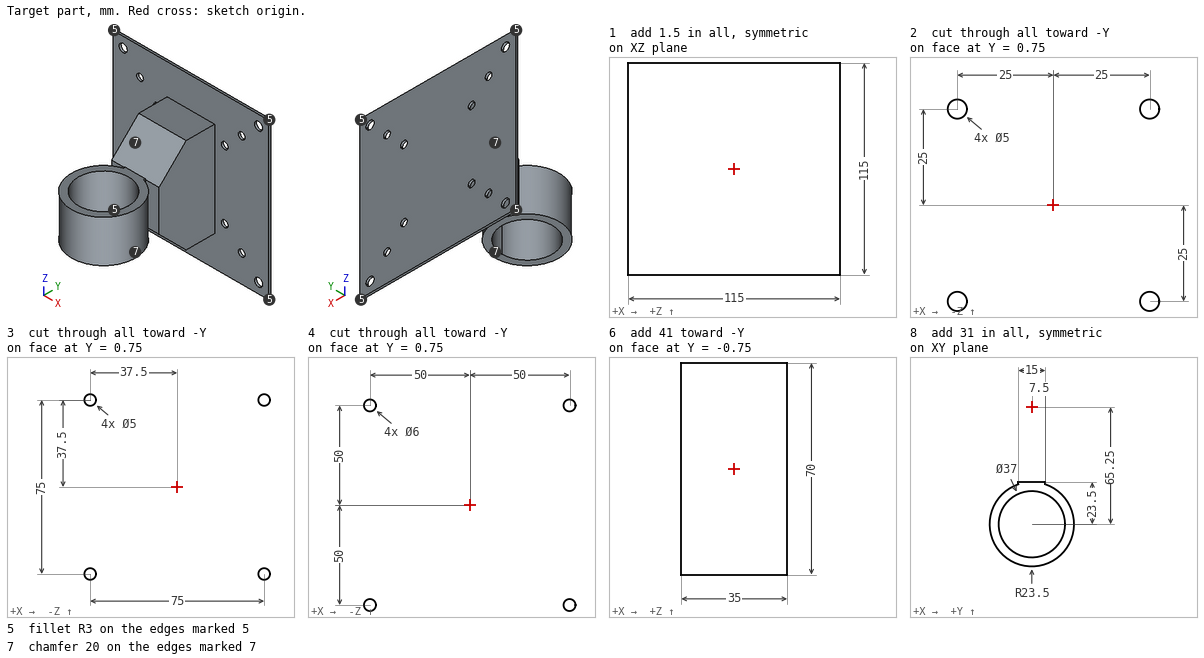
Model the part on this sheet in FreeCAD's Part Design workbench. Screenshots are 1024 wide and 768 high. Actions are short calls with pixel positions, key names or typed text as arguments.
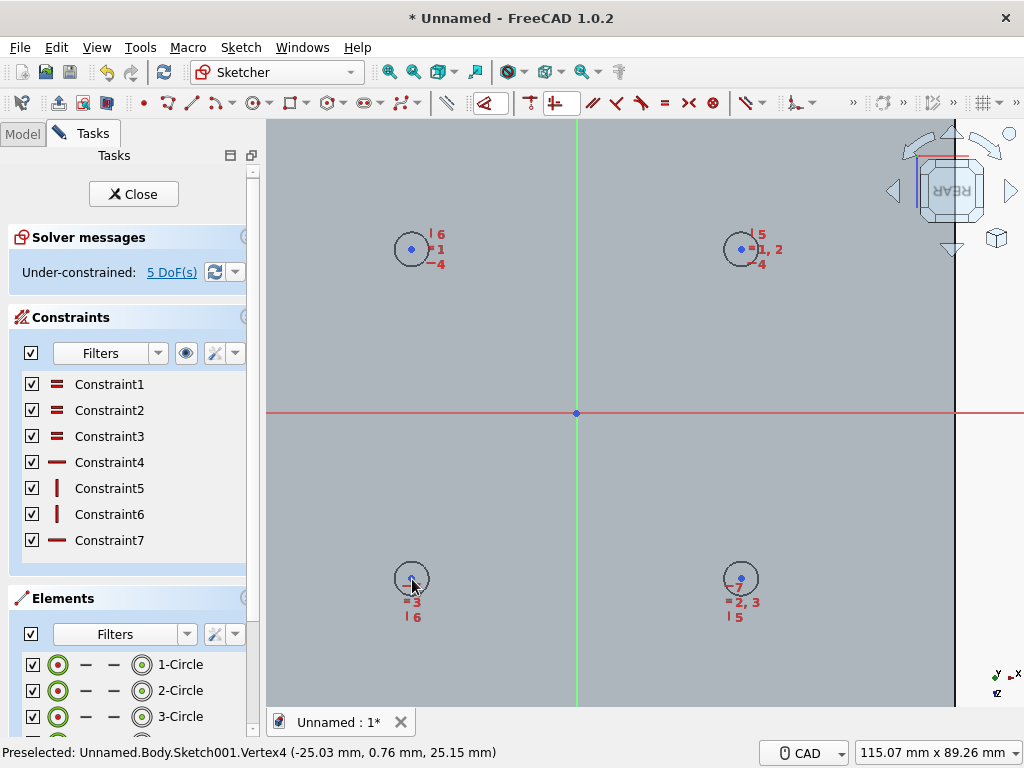
key(d)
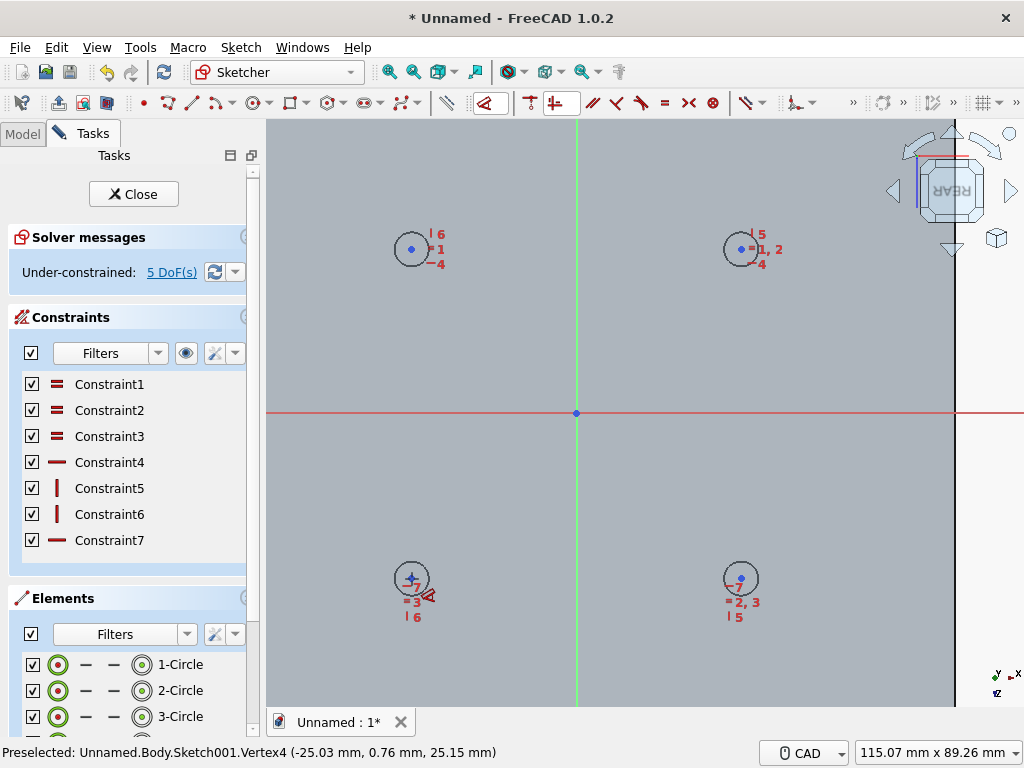
click(424, 237)
click(447, 214)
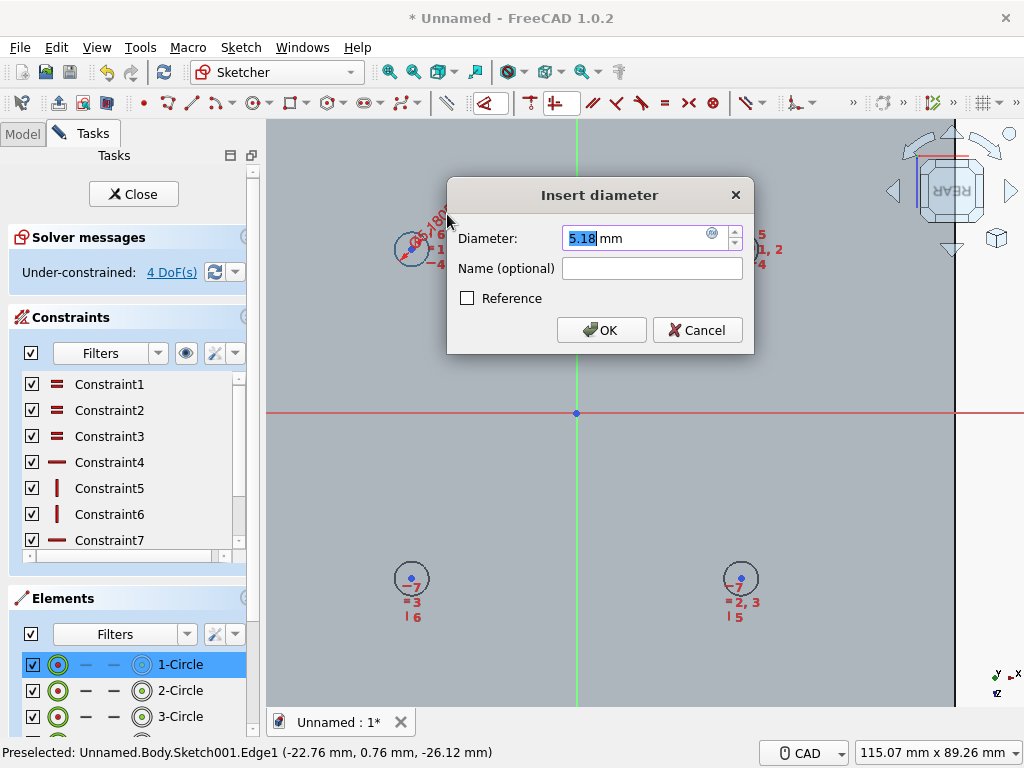
text(5)
key(Return)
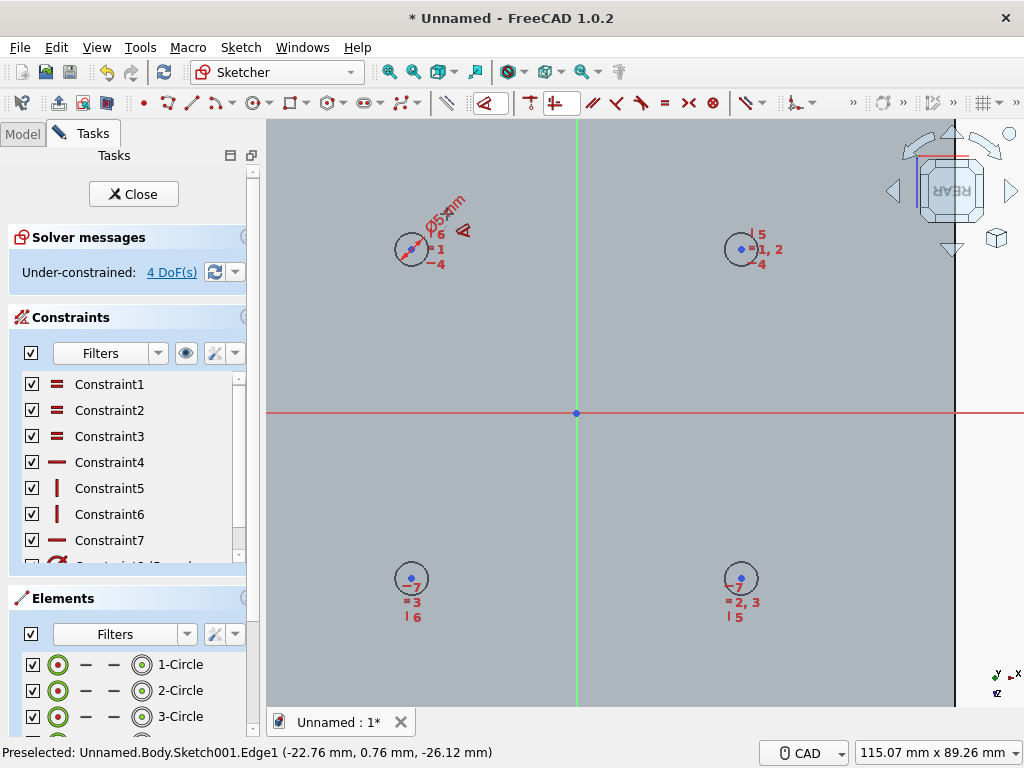
click(412, 249)
click(532, 215)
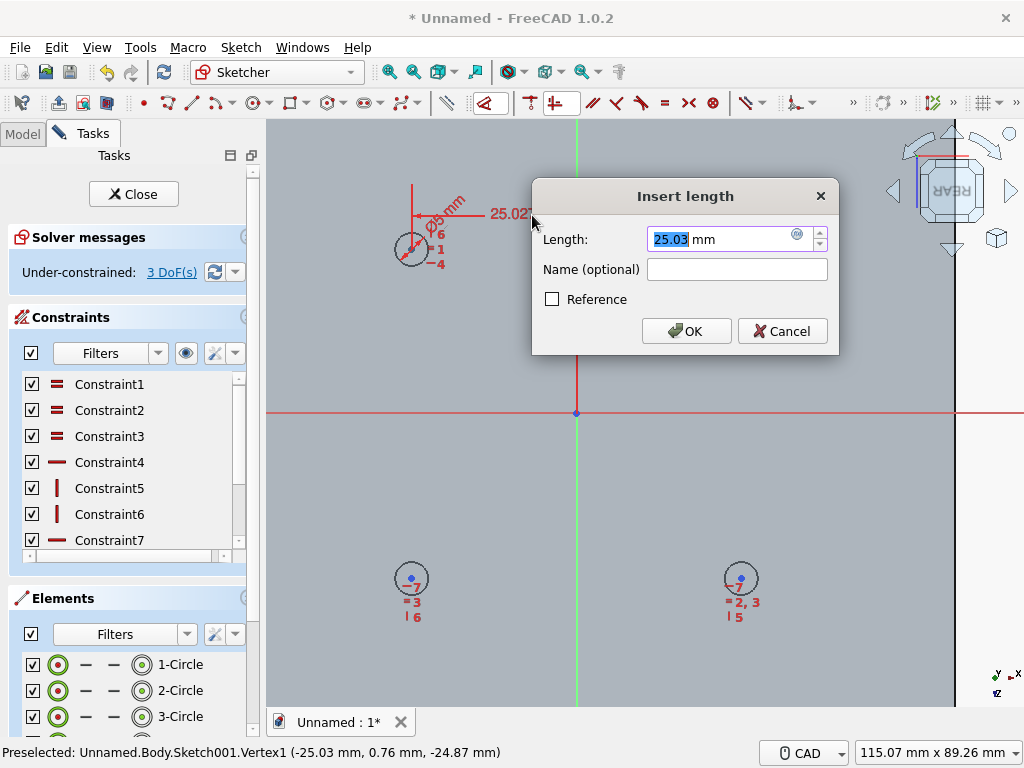
text(25)
key(Return)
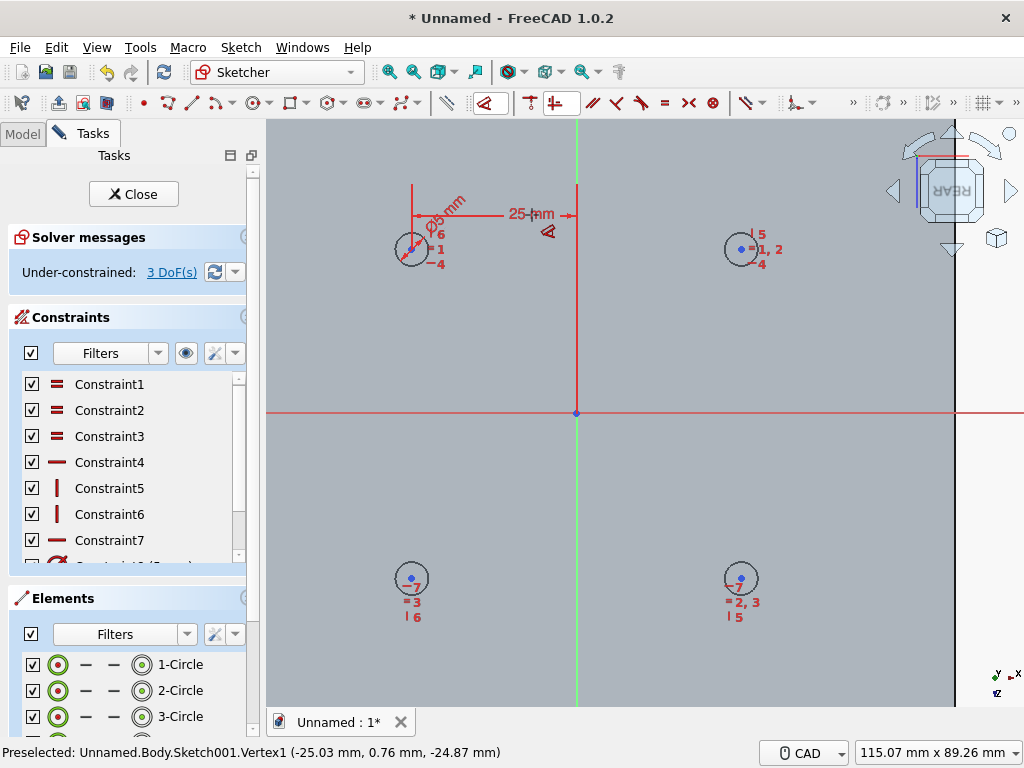
click(412, 249)
click(378, 331)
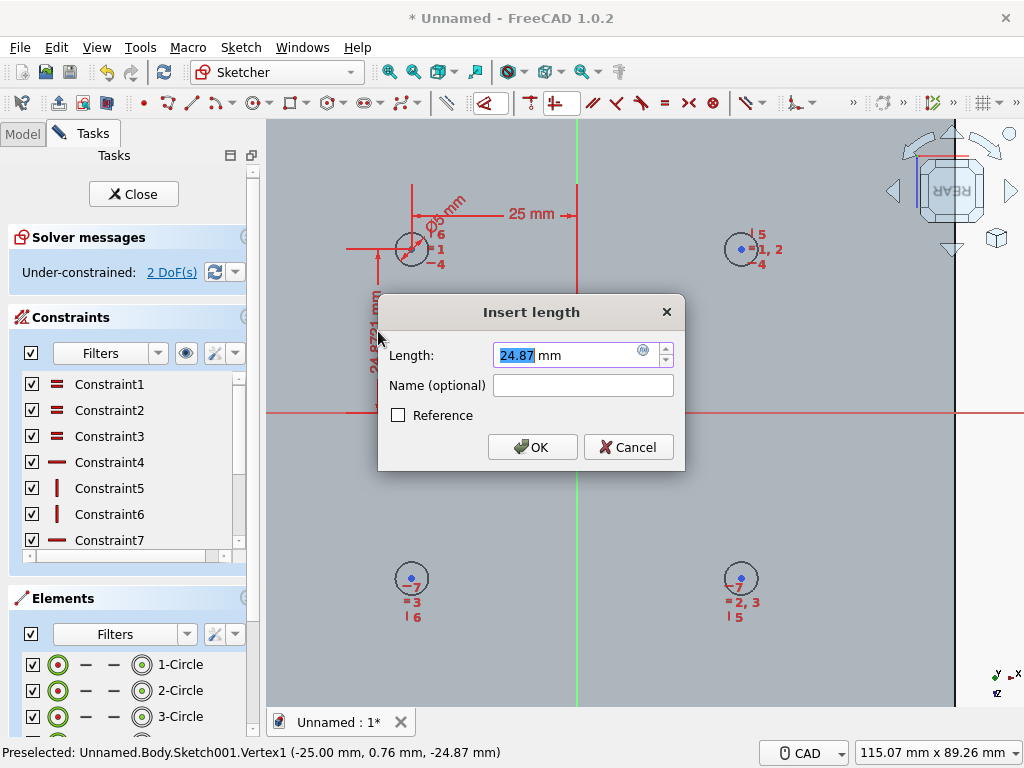
text(25)
key(Return)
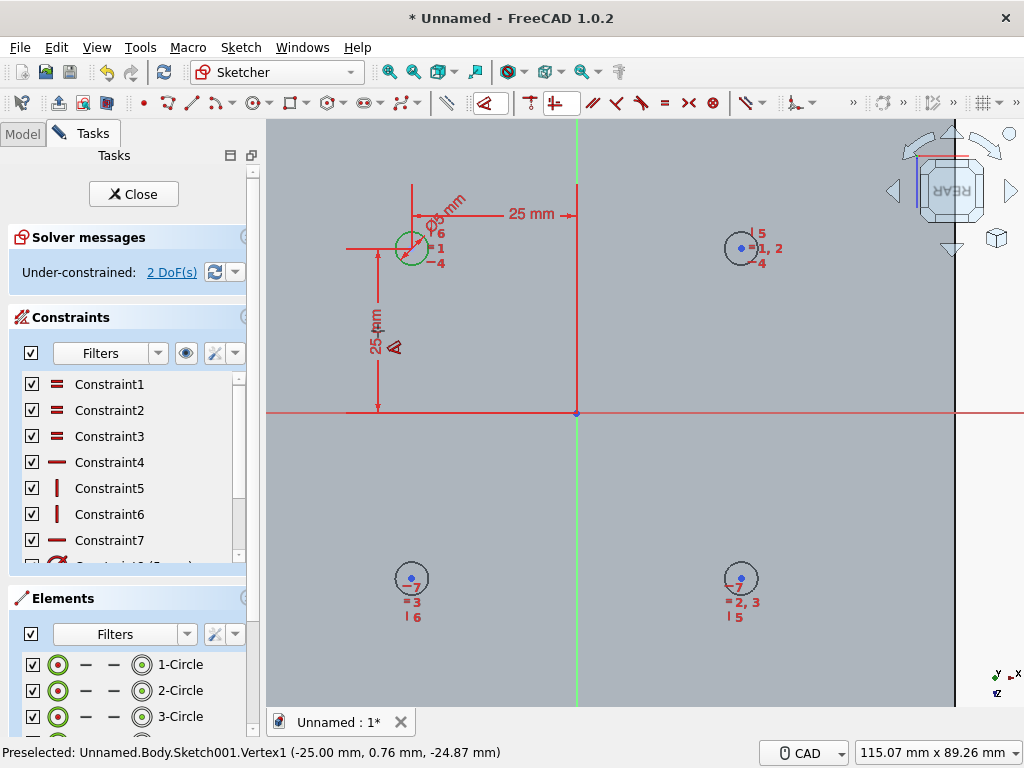
click(741, 249)
click(659, 215)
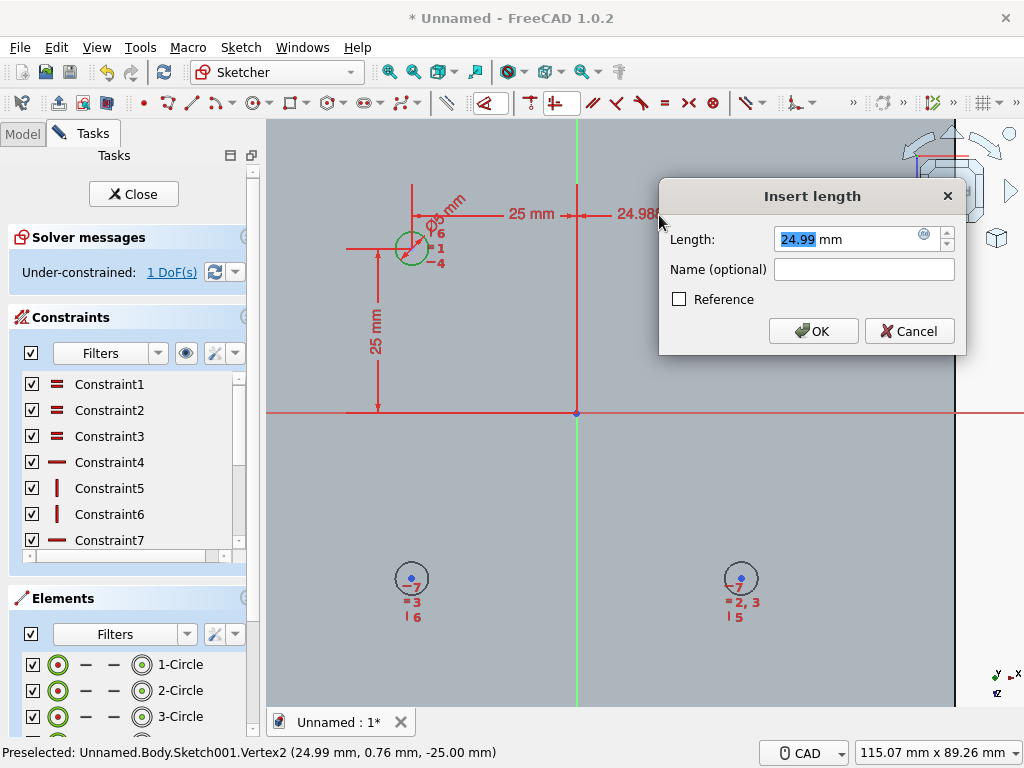
text(25)
key(Return)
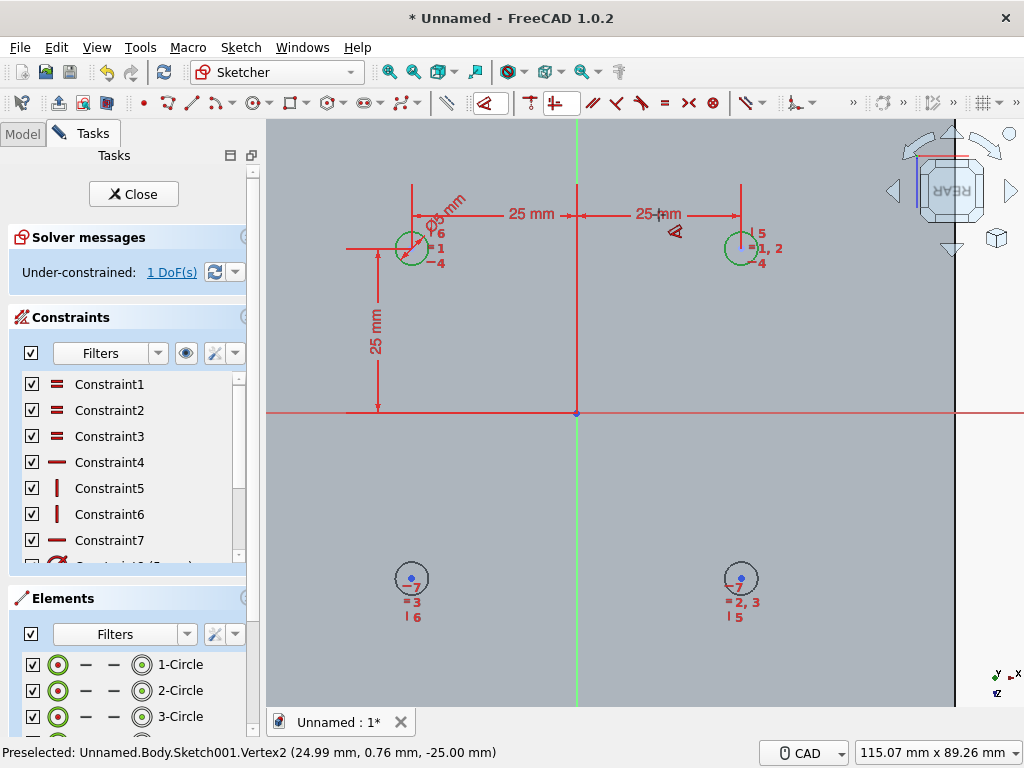
click(741, 579)
click(775, 496)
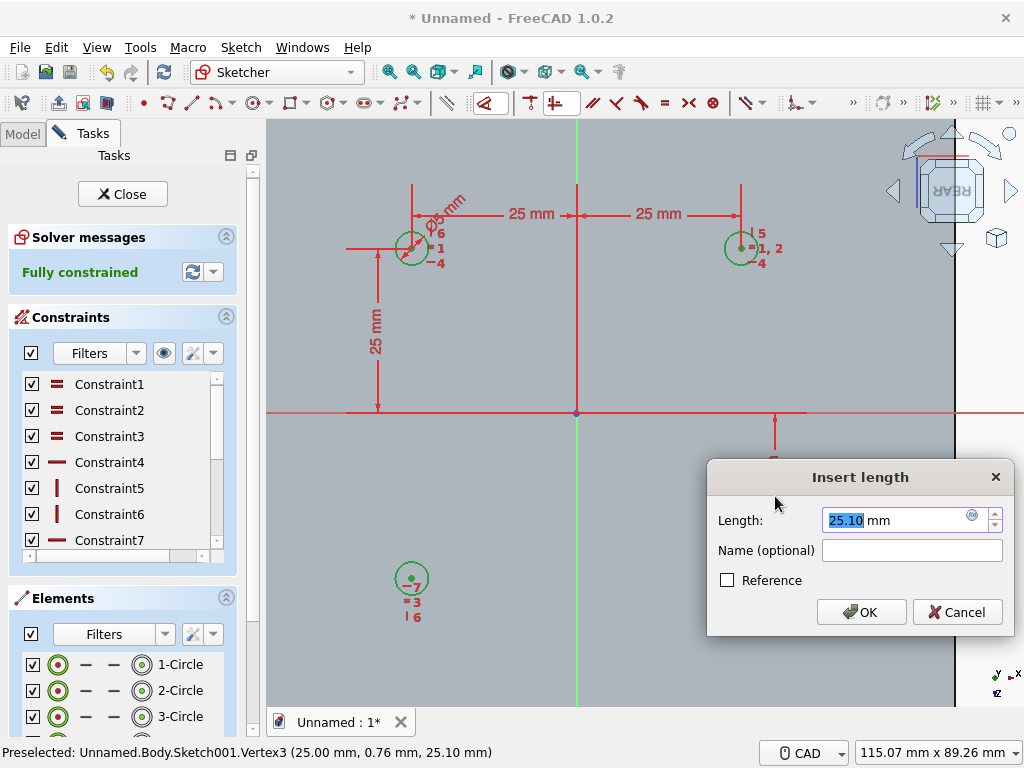
text(25)
key(Return)
key(Escape)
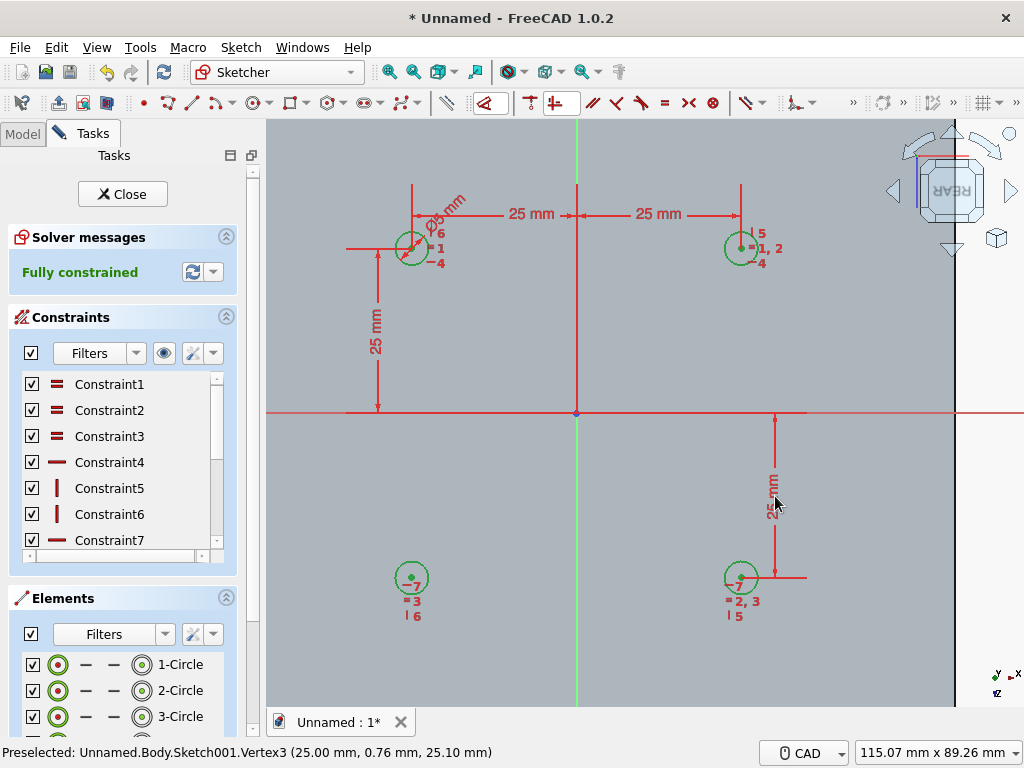
click(123, 194)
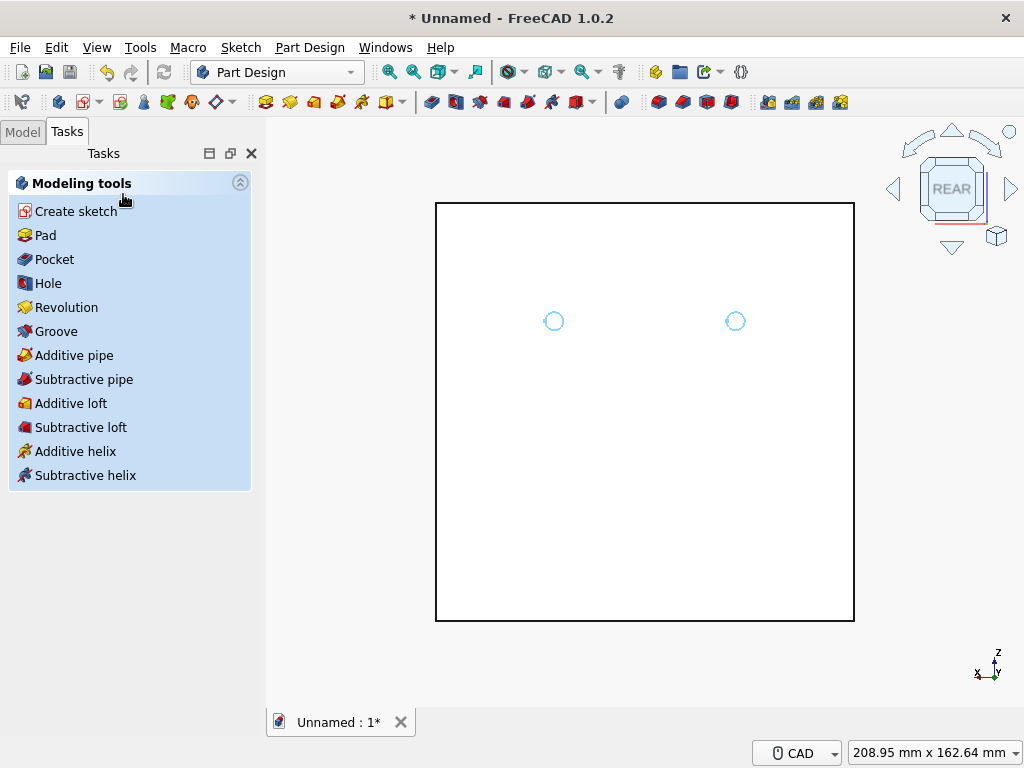
click(432, 102)